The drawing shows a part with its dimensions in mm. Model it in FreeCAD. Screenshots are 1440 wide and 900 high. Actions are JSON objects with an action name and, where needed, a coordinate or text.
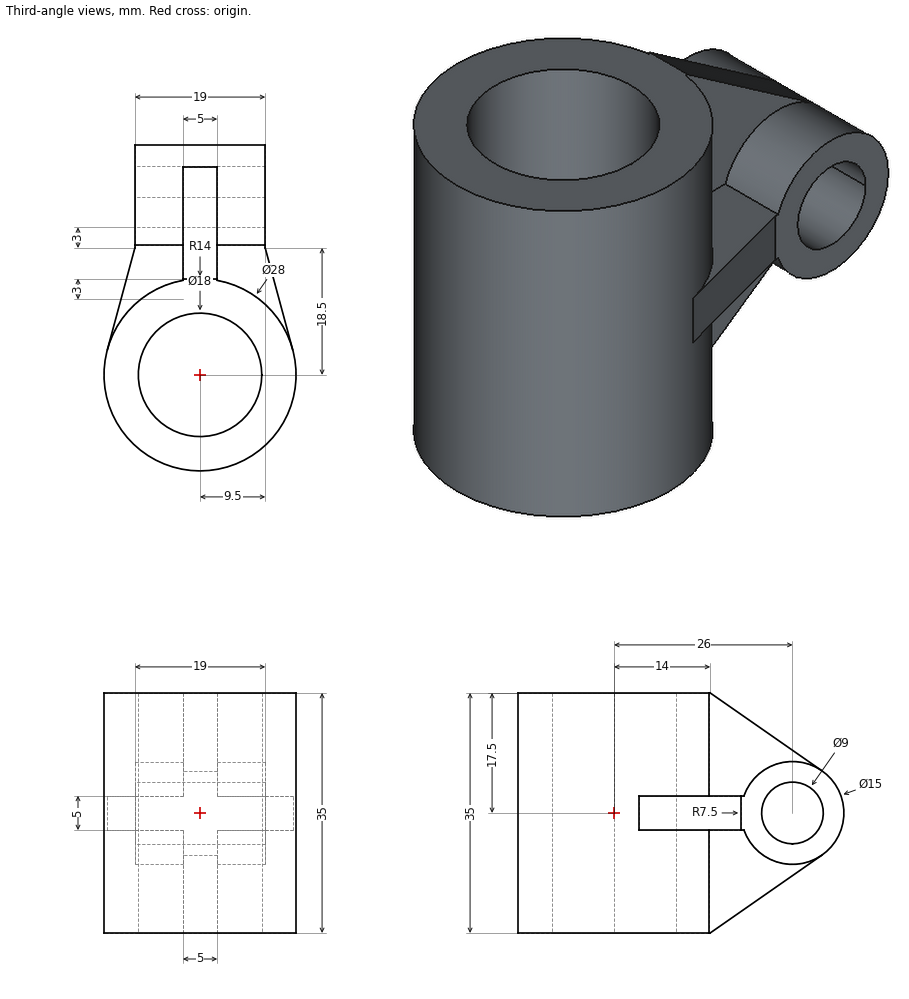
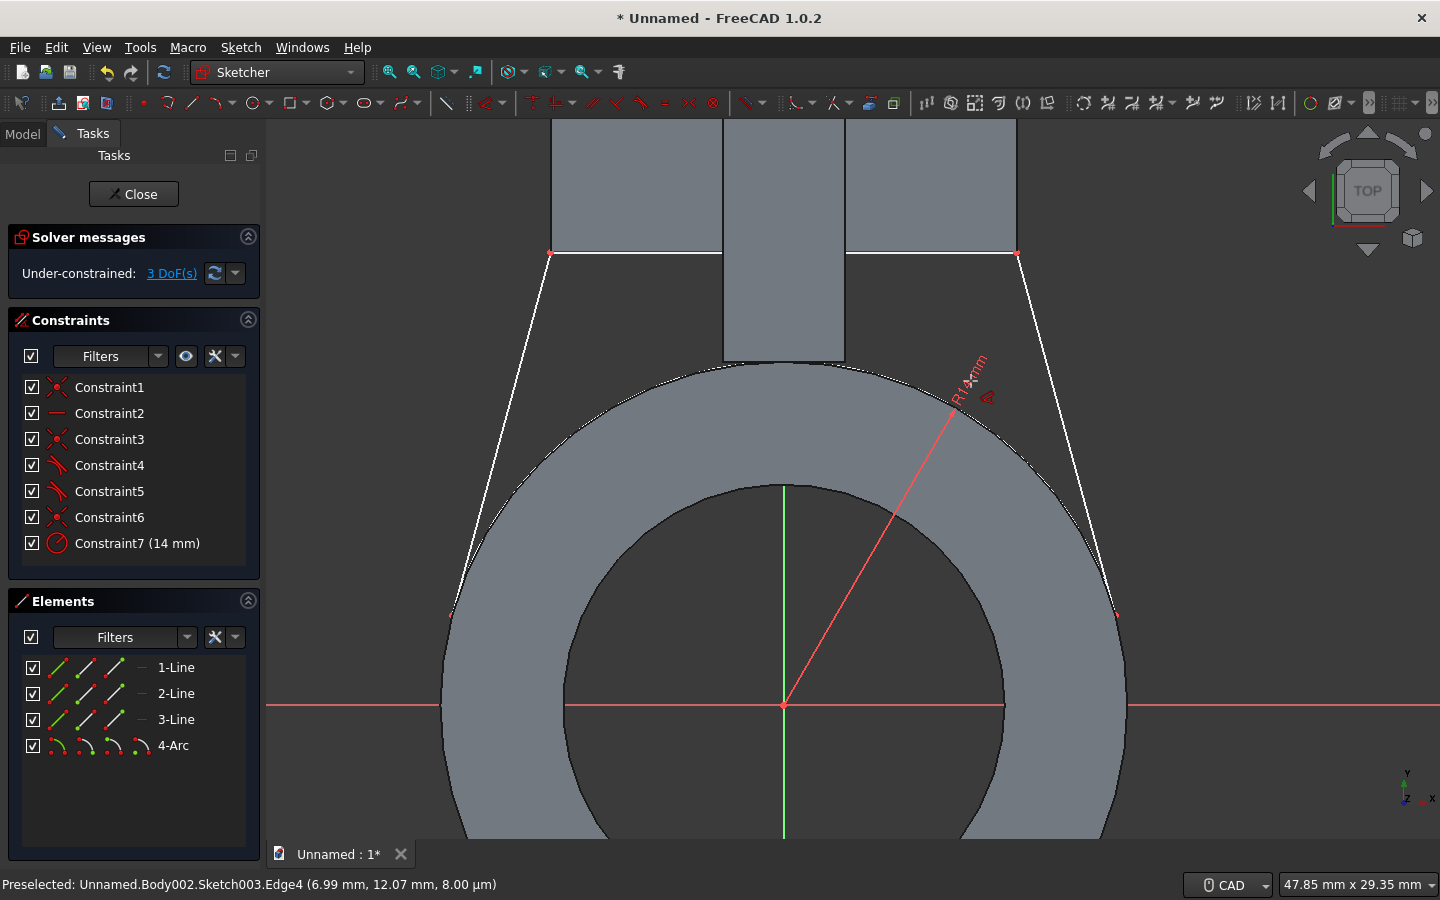
{"action": "left_click", "coordinate": [877, 253]}
{"action": "left_click", "coordinate": [677, 219]}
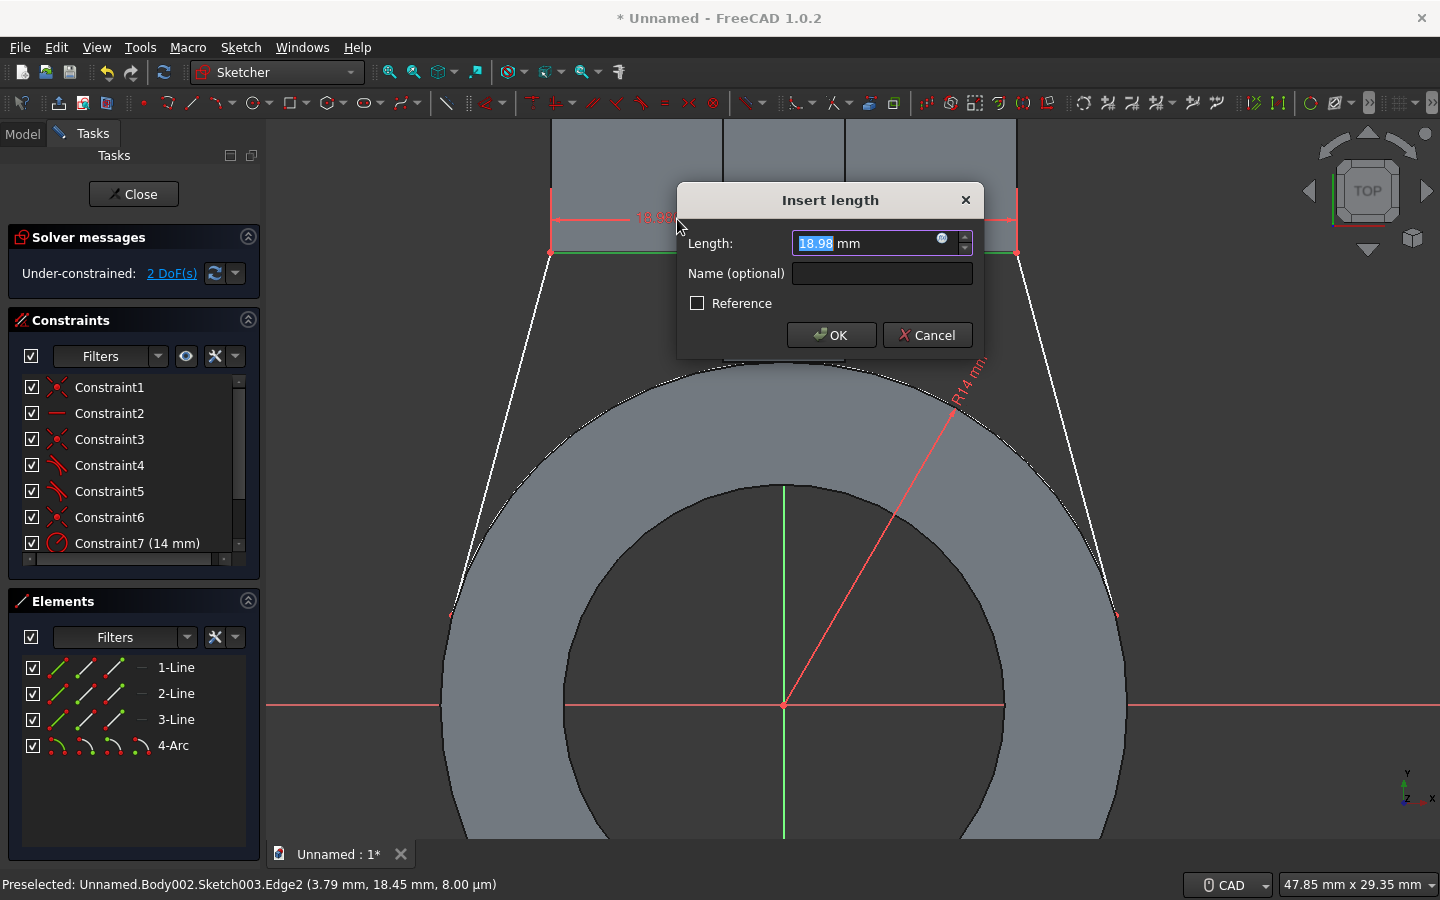
{"action": "type", "text": "19"}
{"action": "key", "text": "Return"}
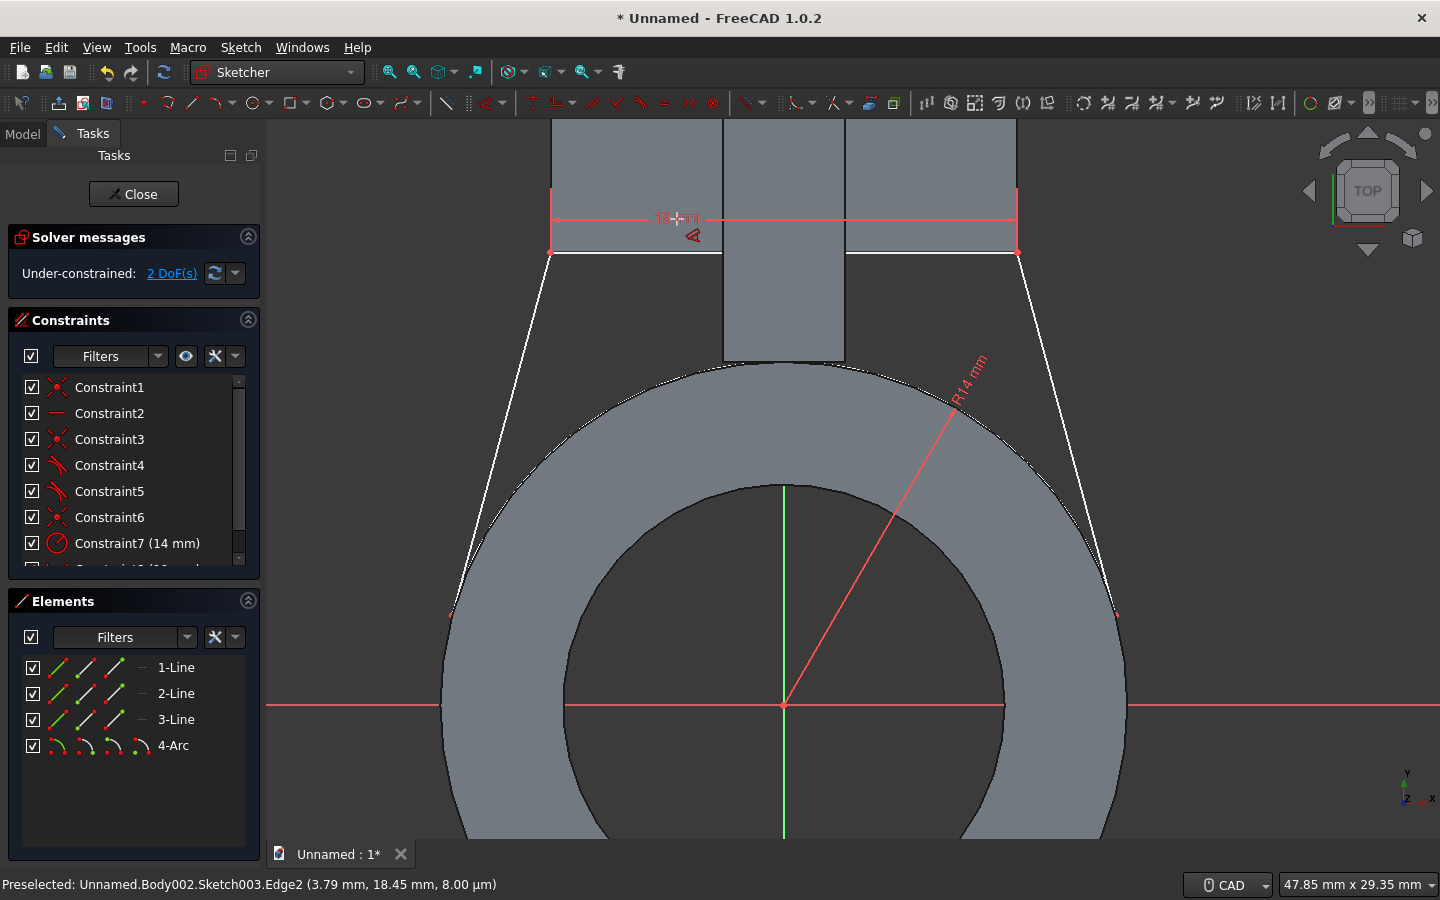
{"action": "left_click", "coordinate": [1017, 253]}
{"action": "left_click", "coordinate": [900, 739]}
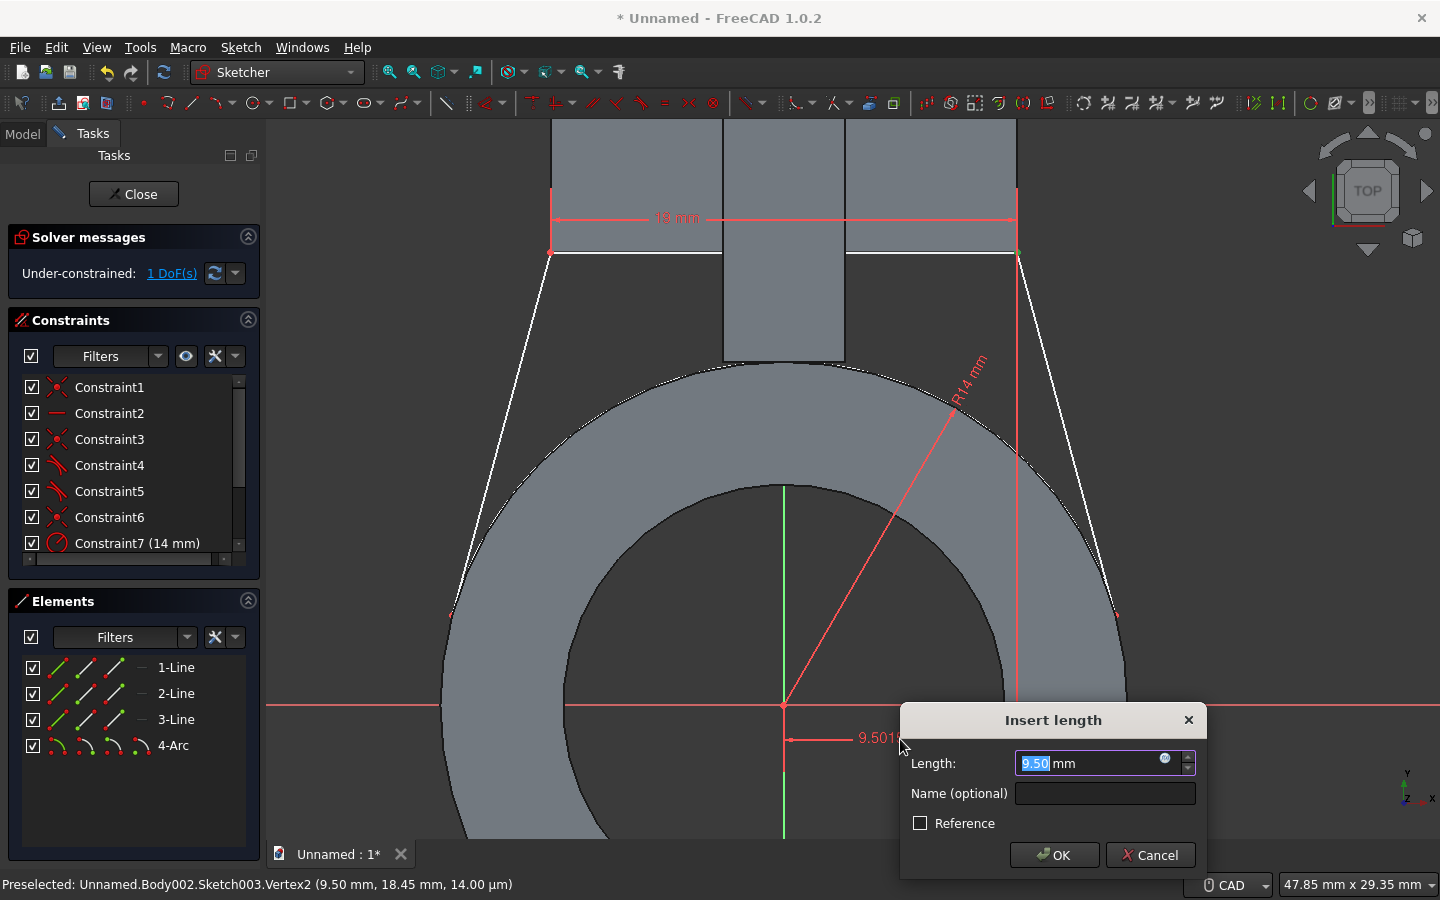
{"action": "type", "text": "9.5"}
{"action": "key", "text": "Return"}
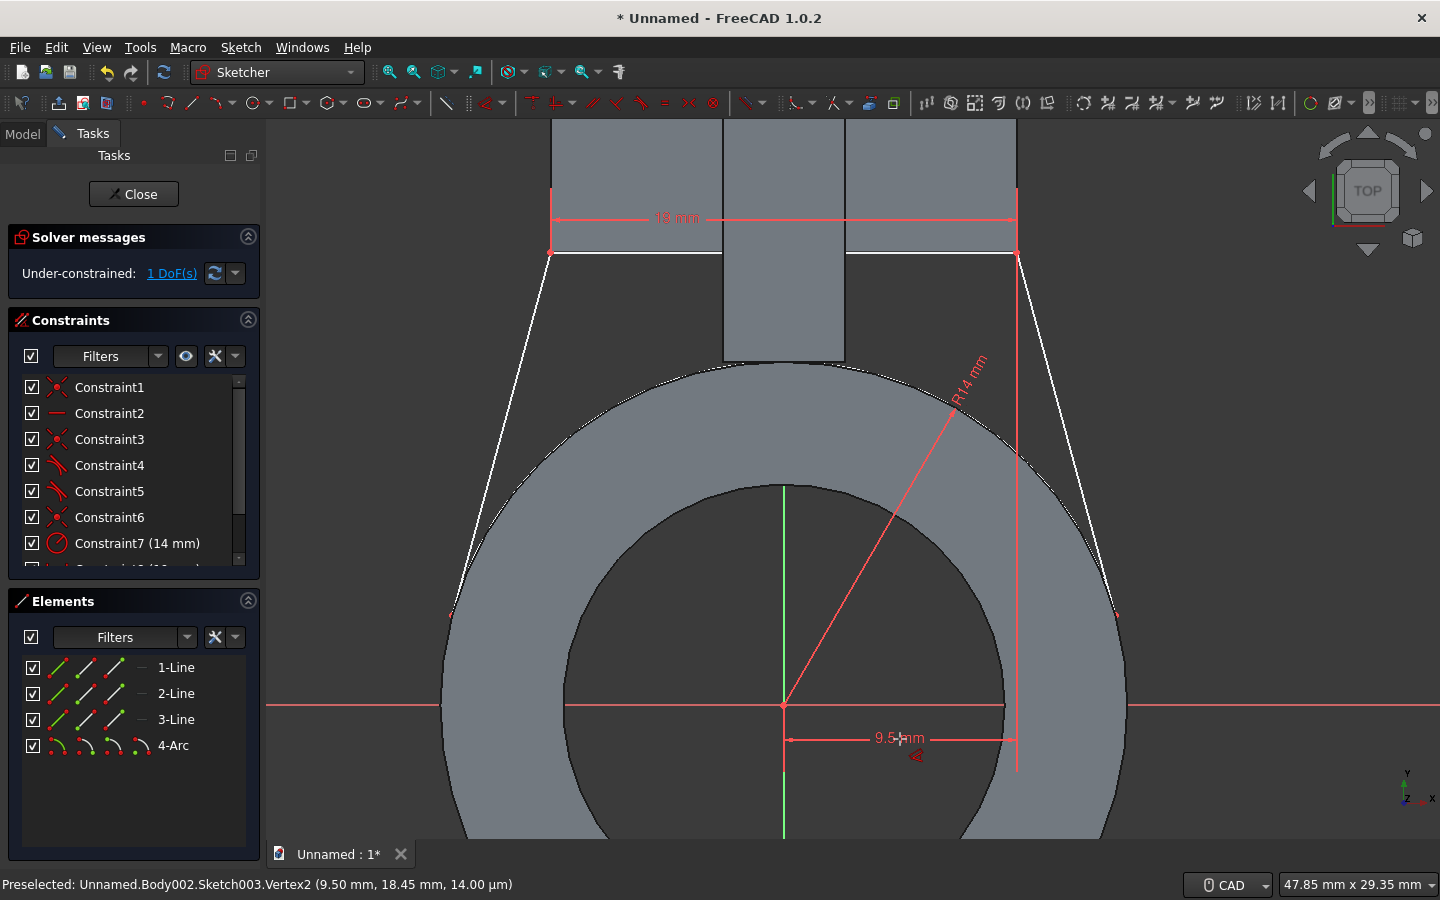
{"action": "left_click", "coordinate": [1017, 253]}
{"action": "left_click", "coordinate": [1051, 583]}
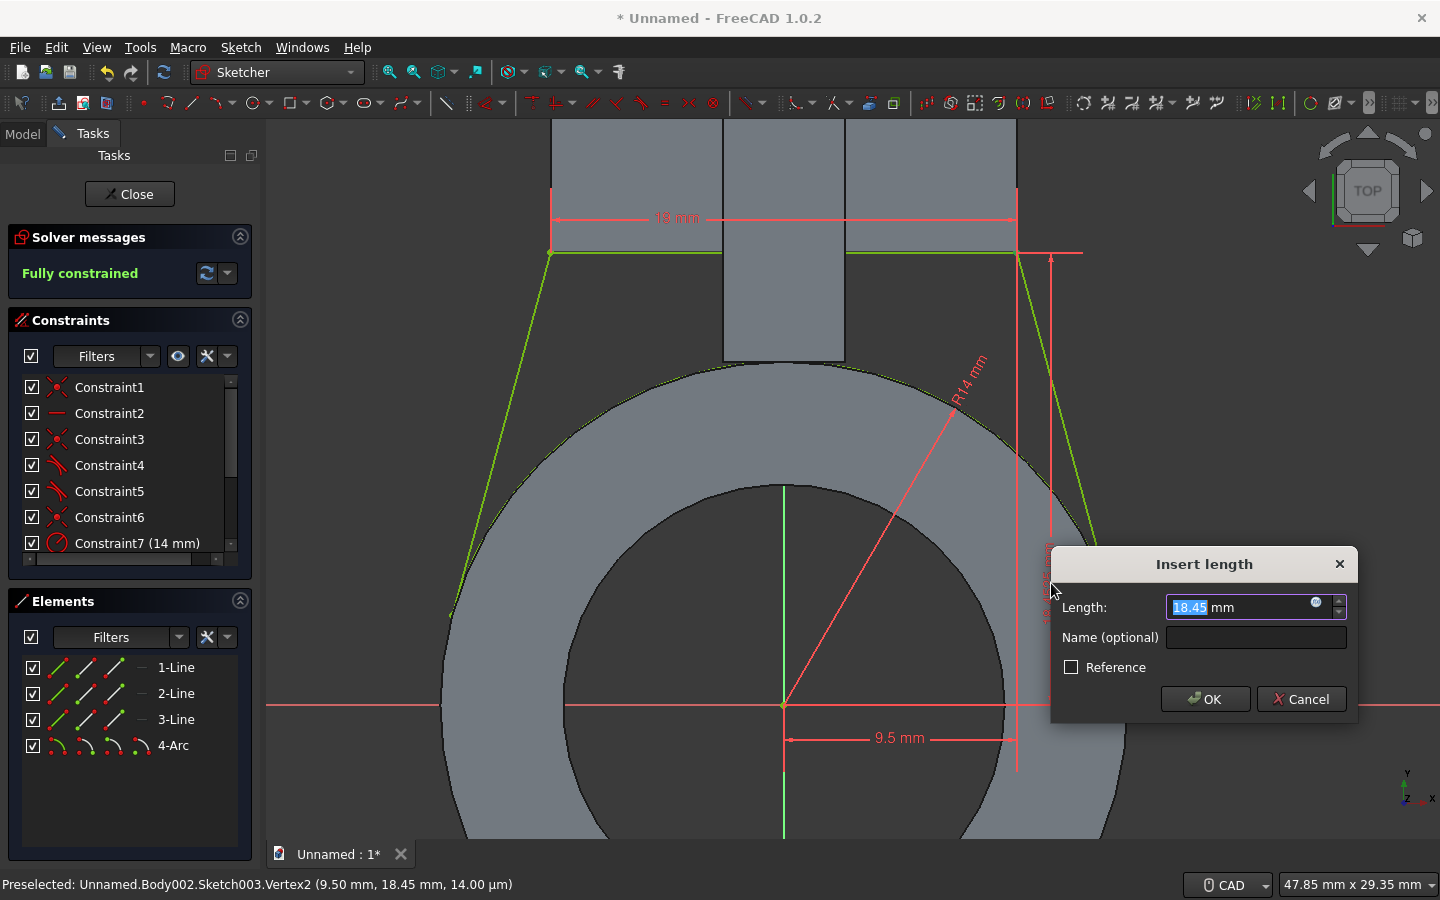
{"action": "type", "text": "18.5"}
{"action": "key", "text": "Return"}
{"action": "key", "text": "Escape"}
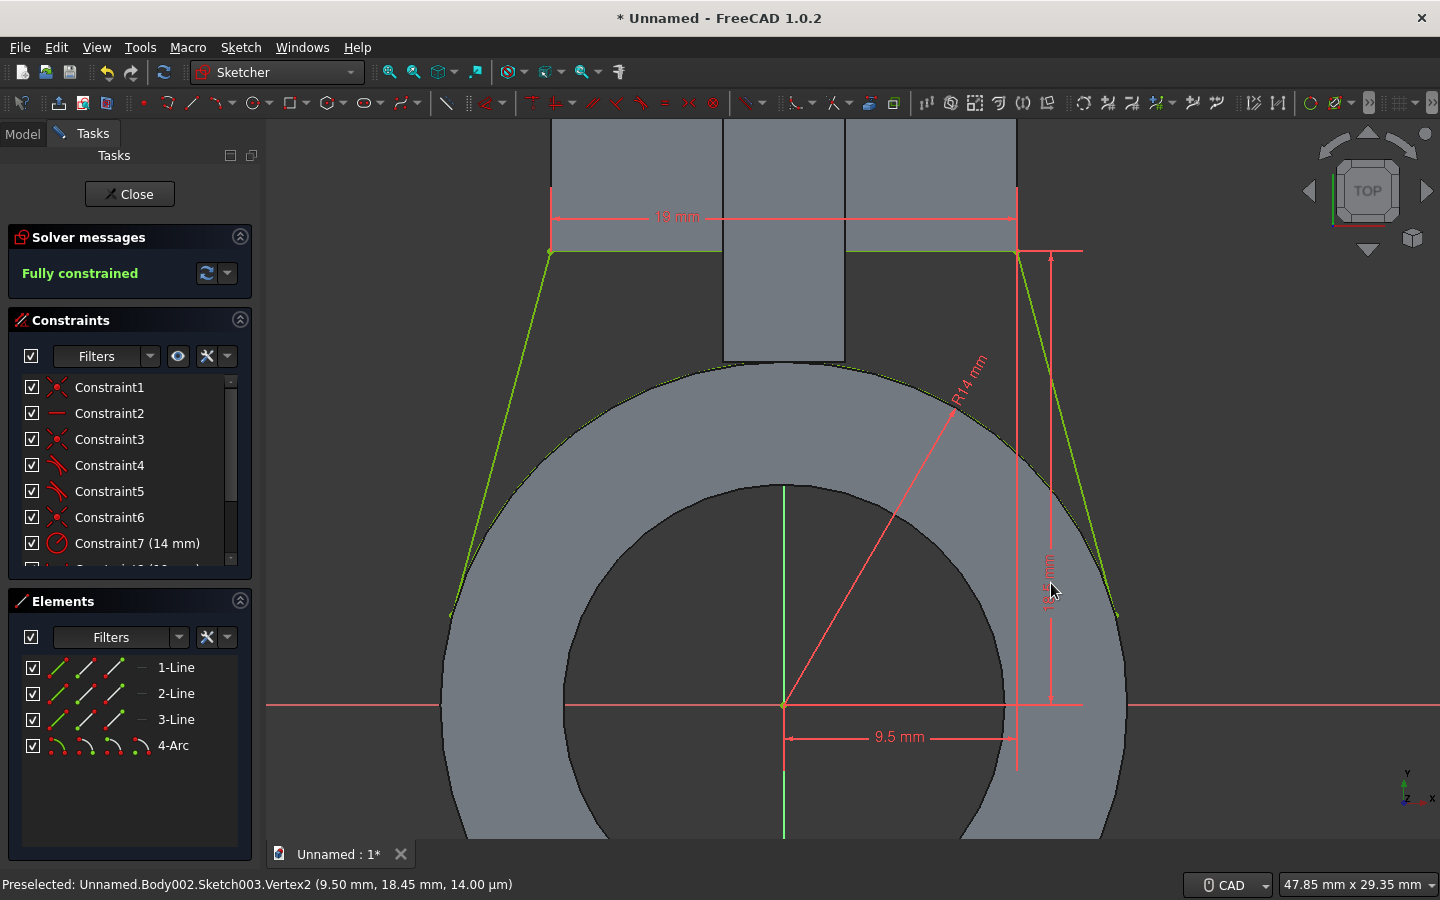
{"action": "left_click", "coordinate": [130, 194]}